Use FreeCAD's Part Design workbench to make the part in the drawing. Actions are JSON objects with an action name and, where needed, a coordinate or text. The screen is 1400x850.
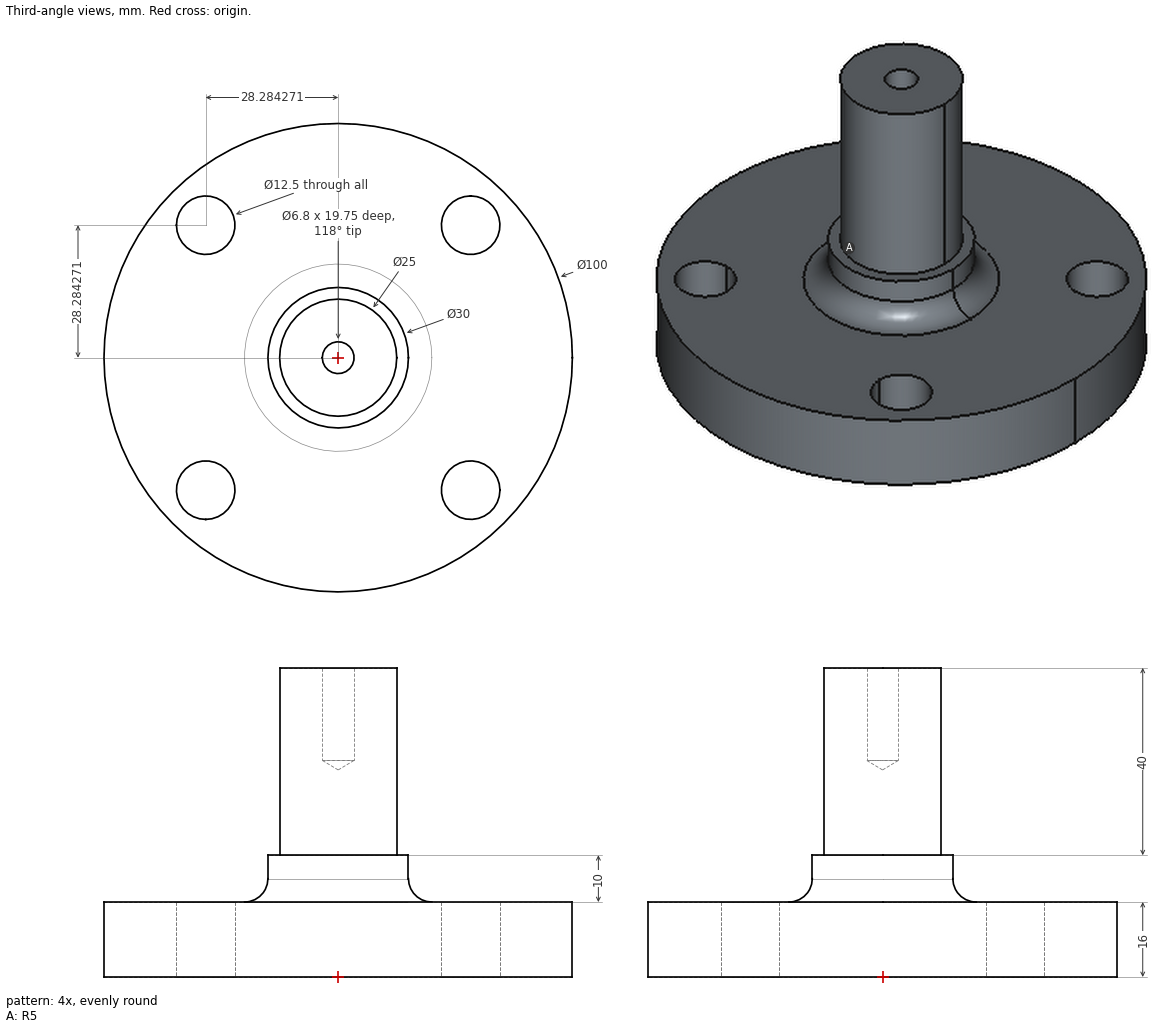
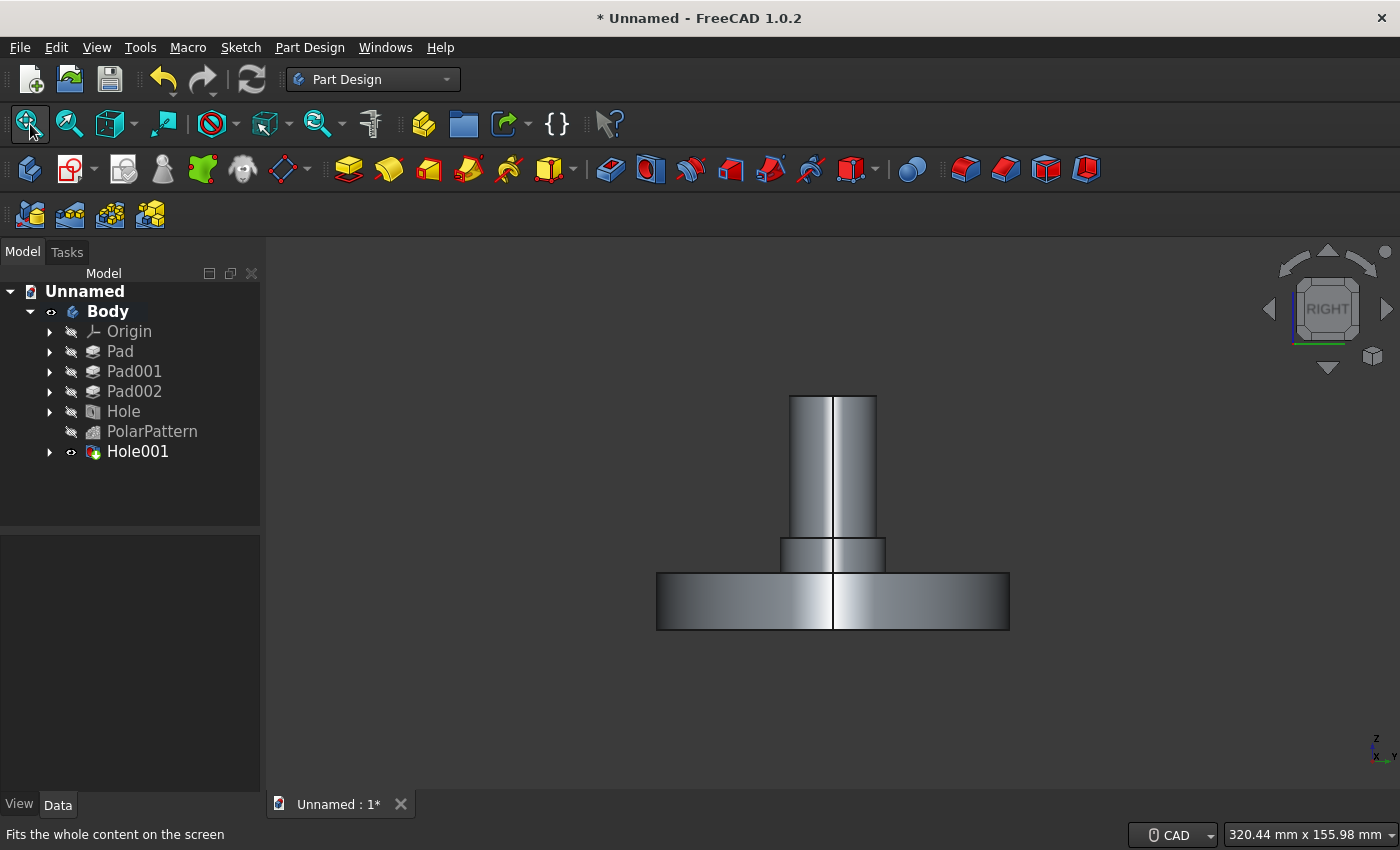
{"action": "left_click", "coordinate": [30, 124]}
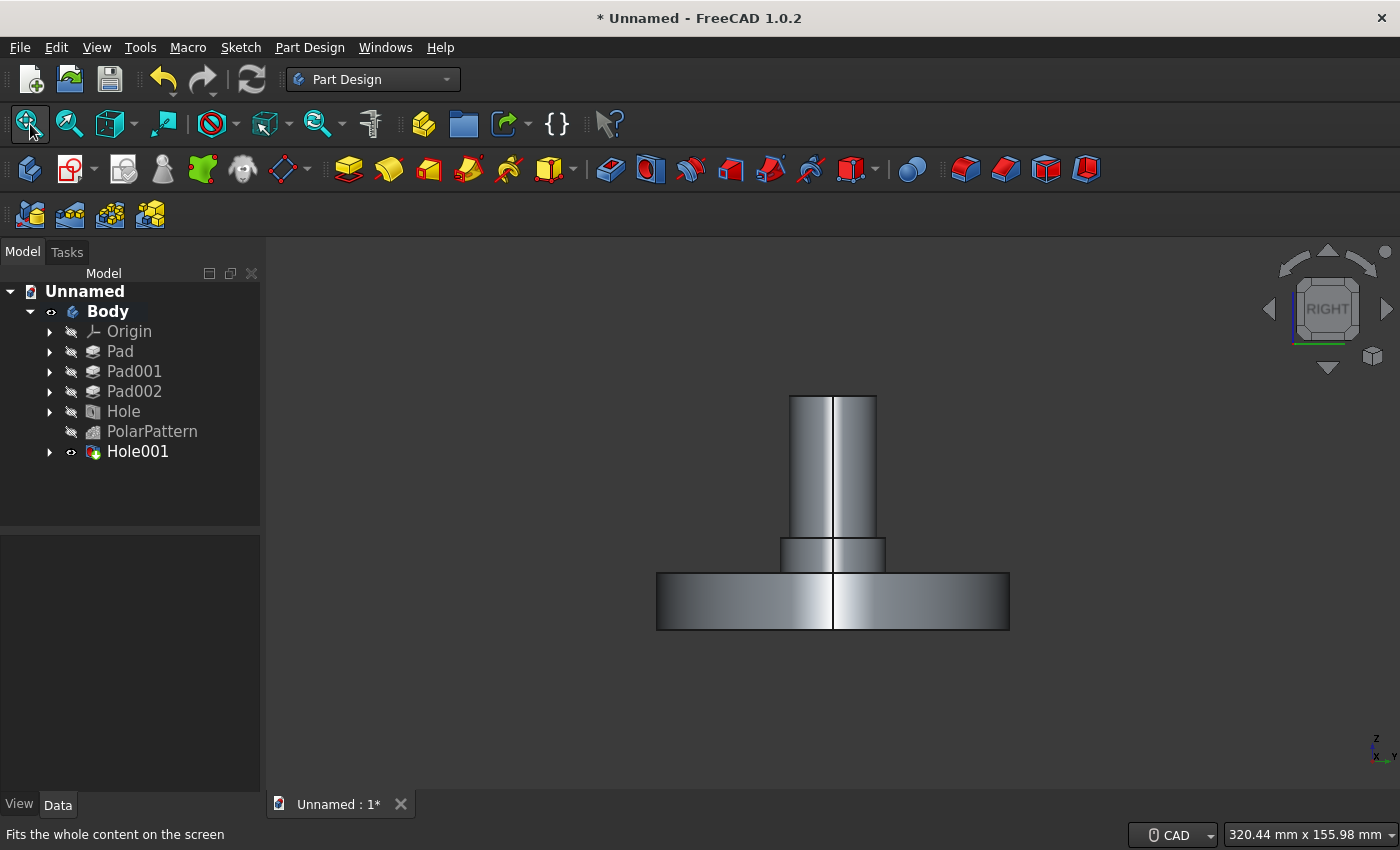
{"action": "key", "text": "5"}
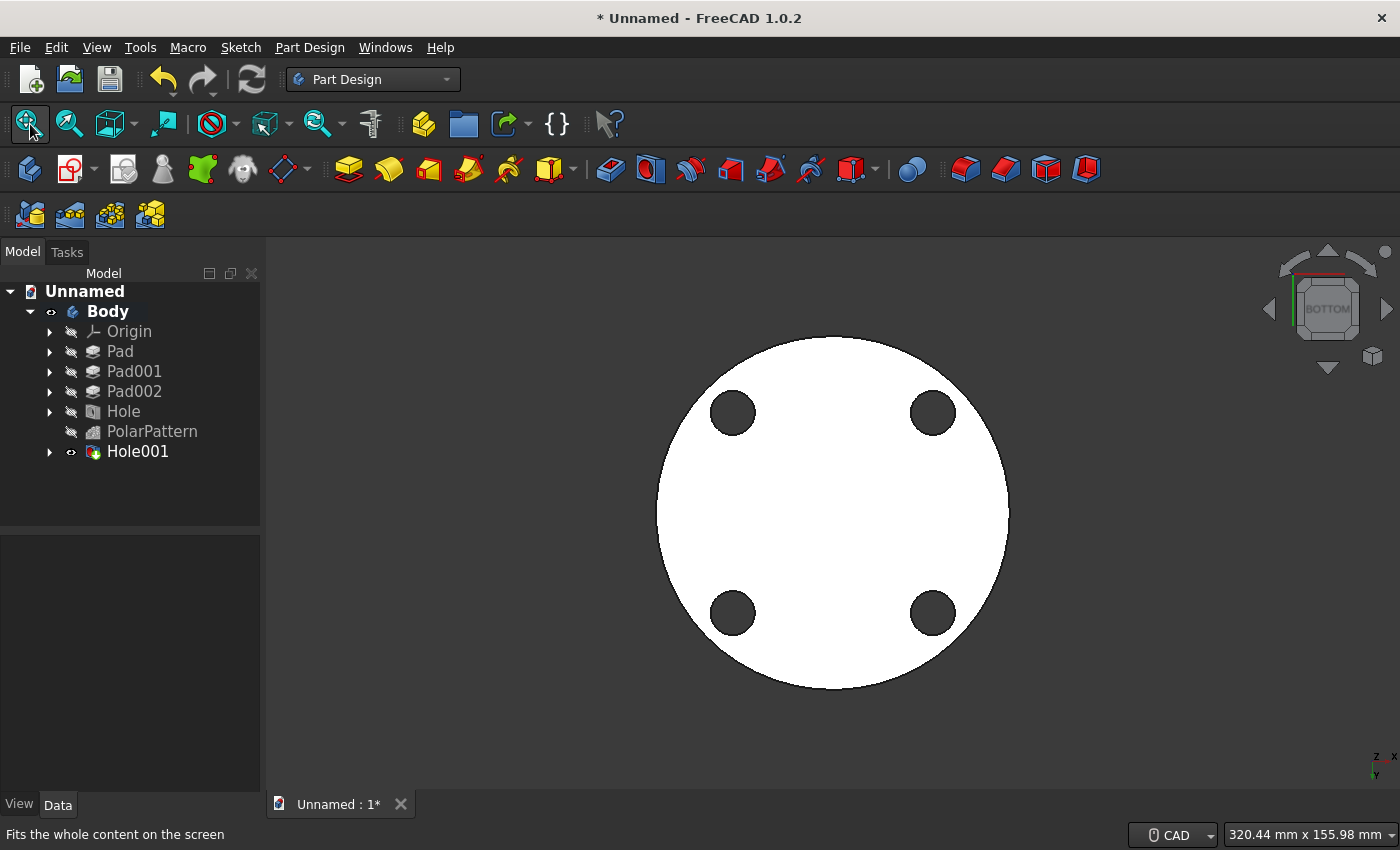
{"action": "key", "text": "4"}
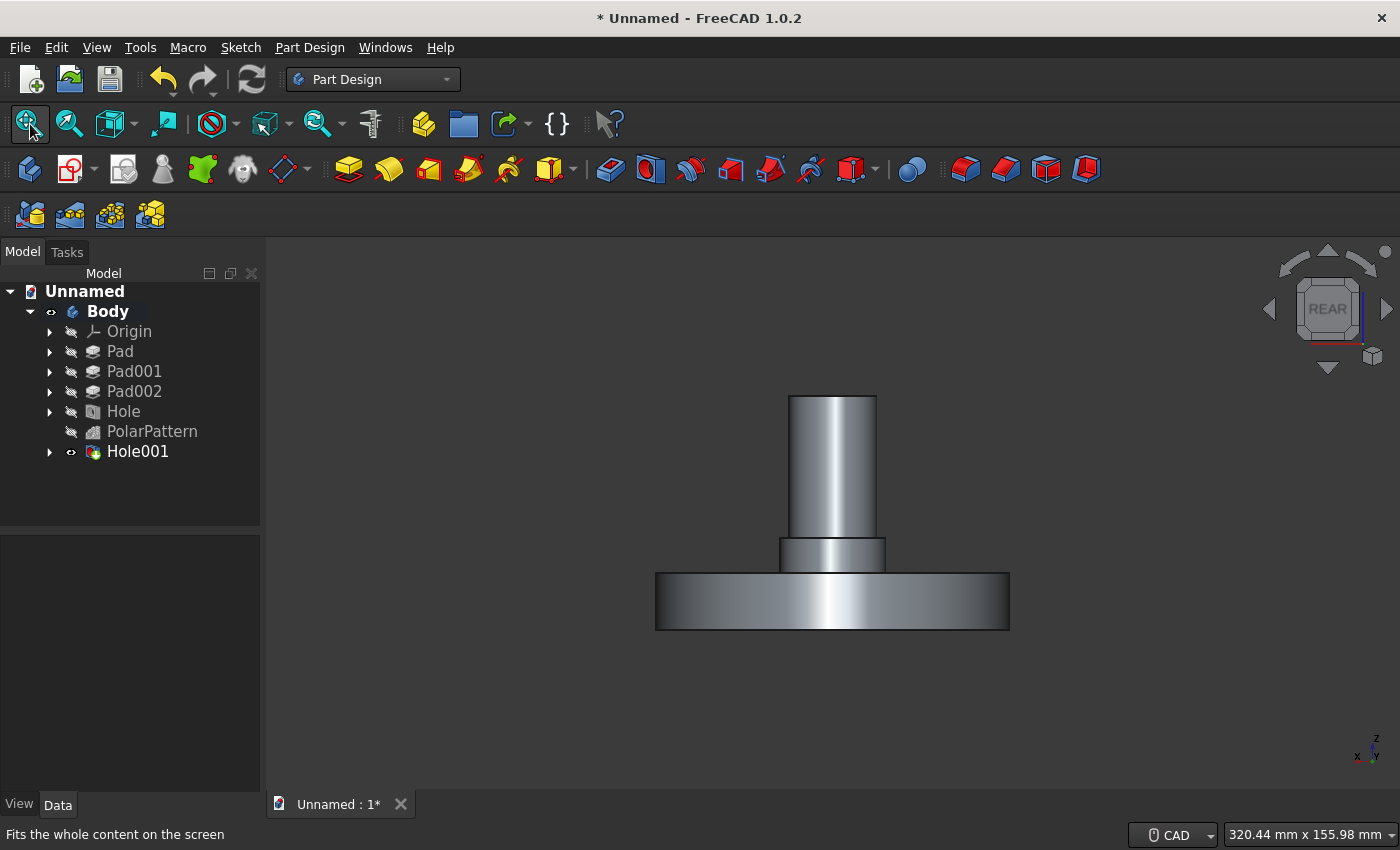
{"action": "left_click", "coordinate": [30, 124]}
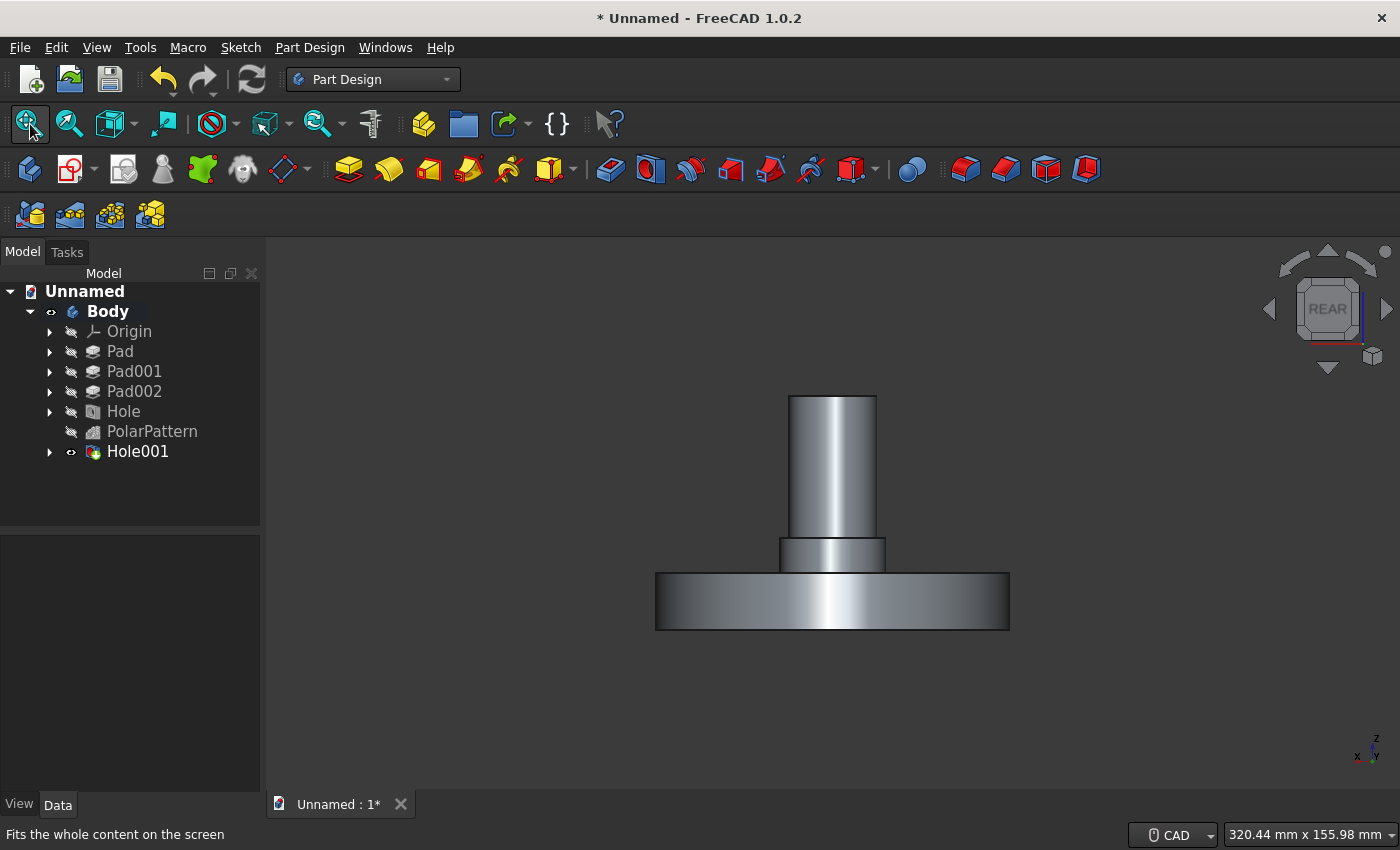
{"action": "key", "text": "6"}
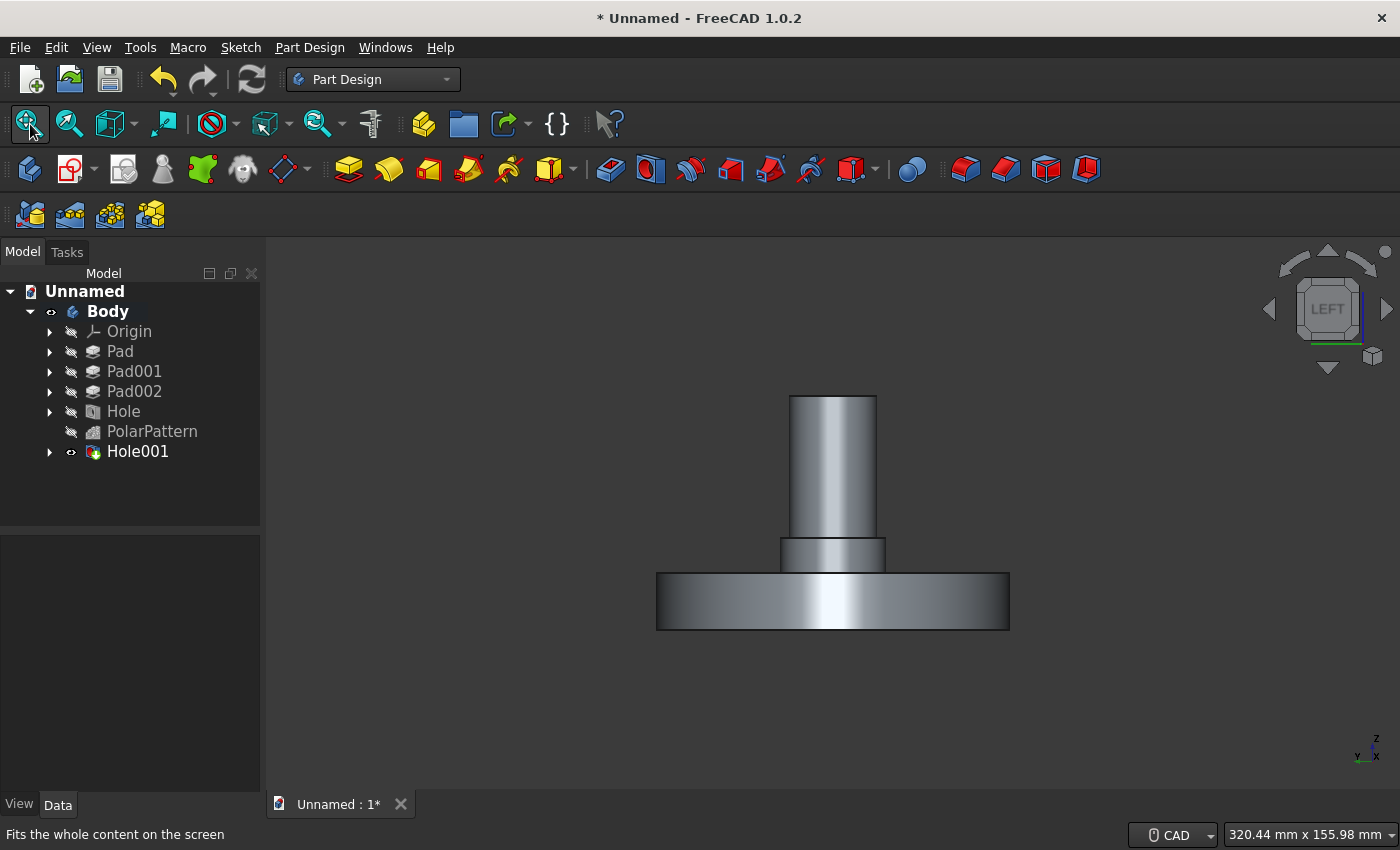
{"action": "key", "text": "v f"}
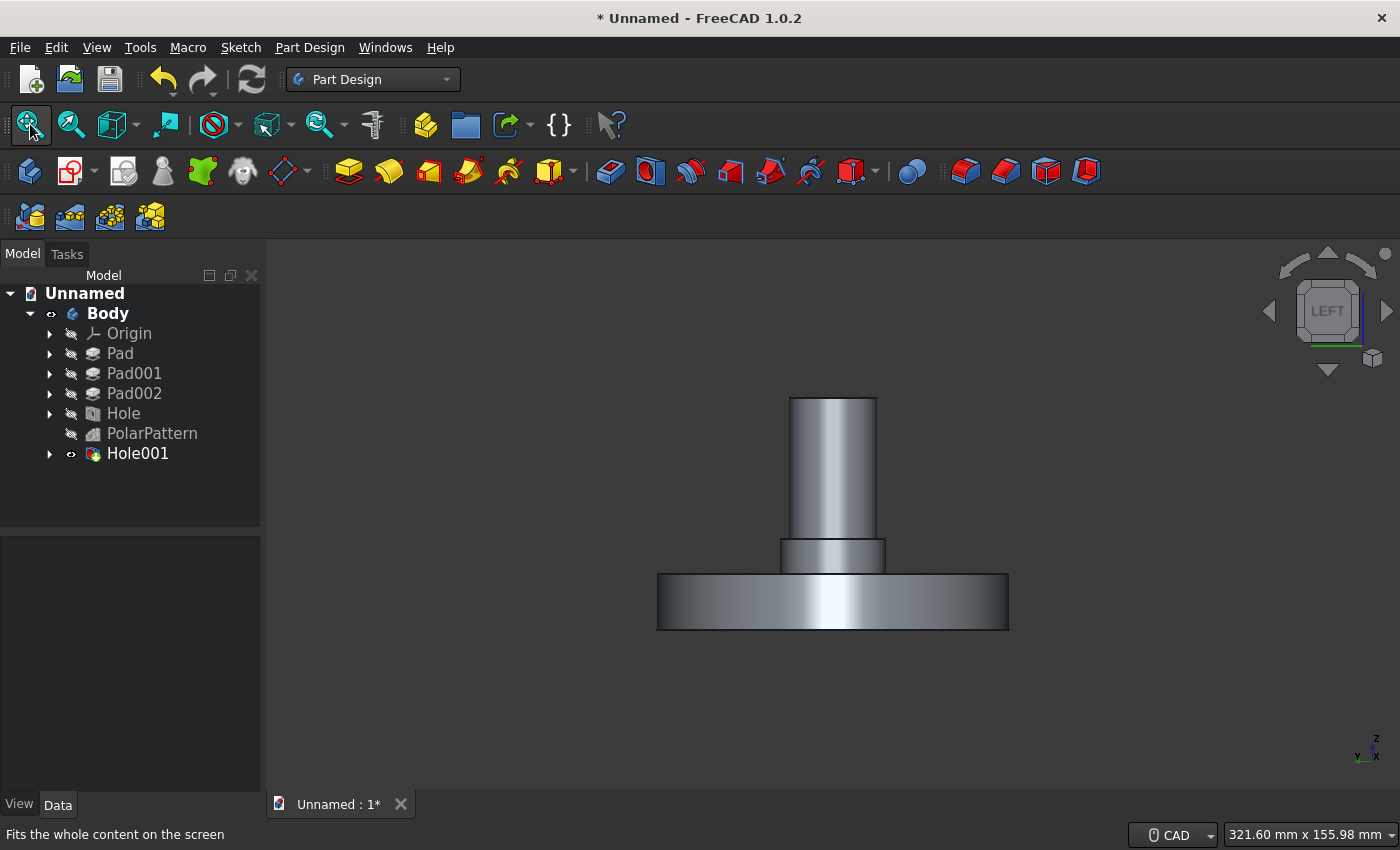
{"action": "key", "text": "v 3"}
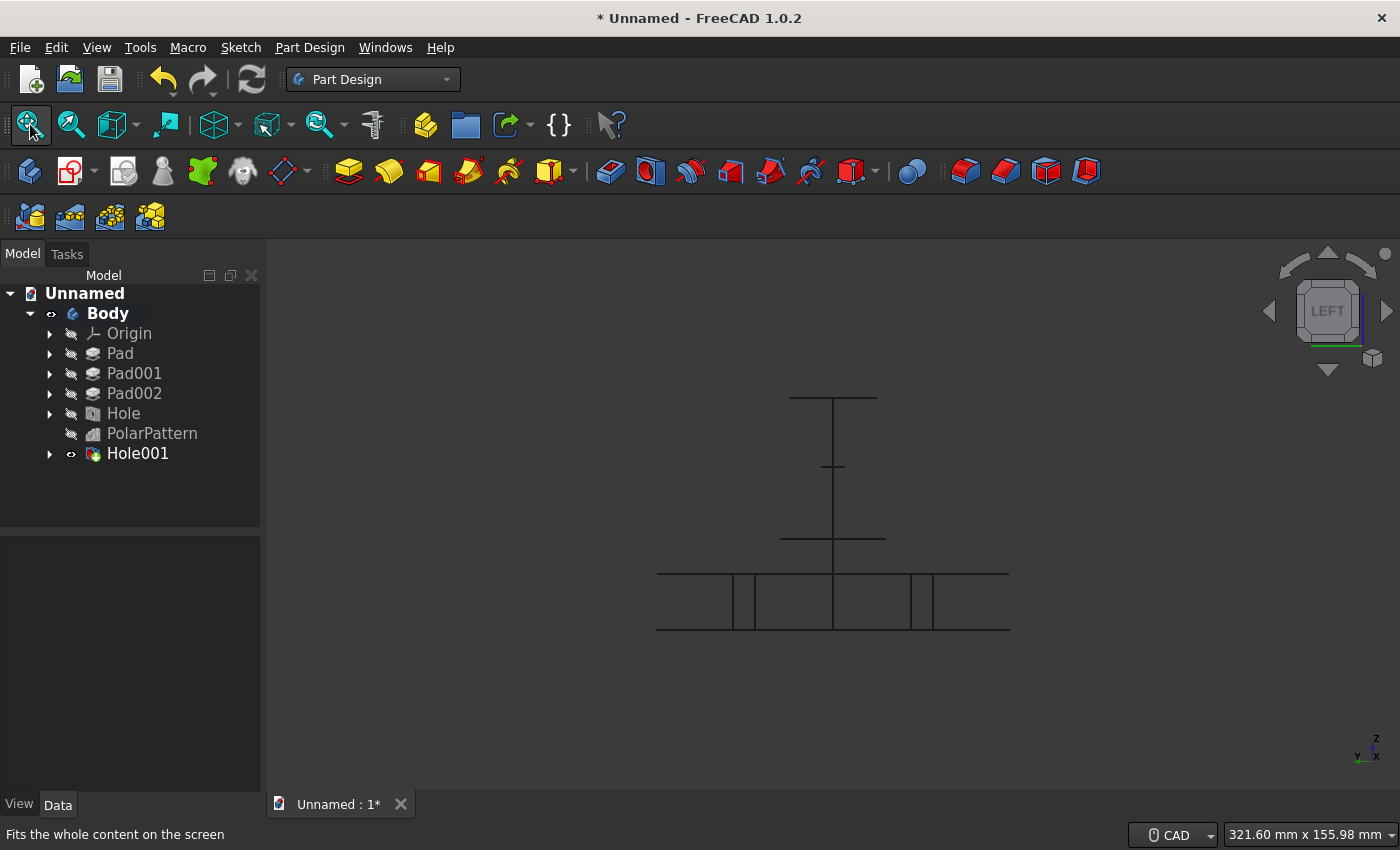
{"action": "key", "text": "0"}